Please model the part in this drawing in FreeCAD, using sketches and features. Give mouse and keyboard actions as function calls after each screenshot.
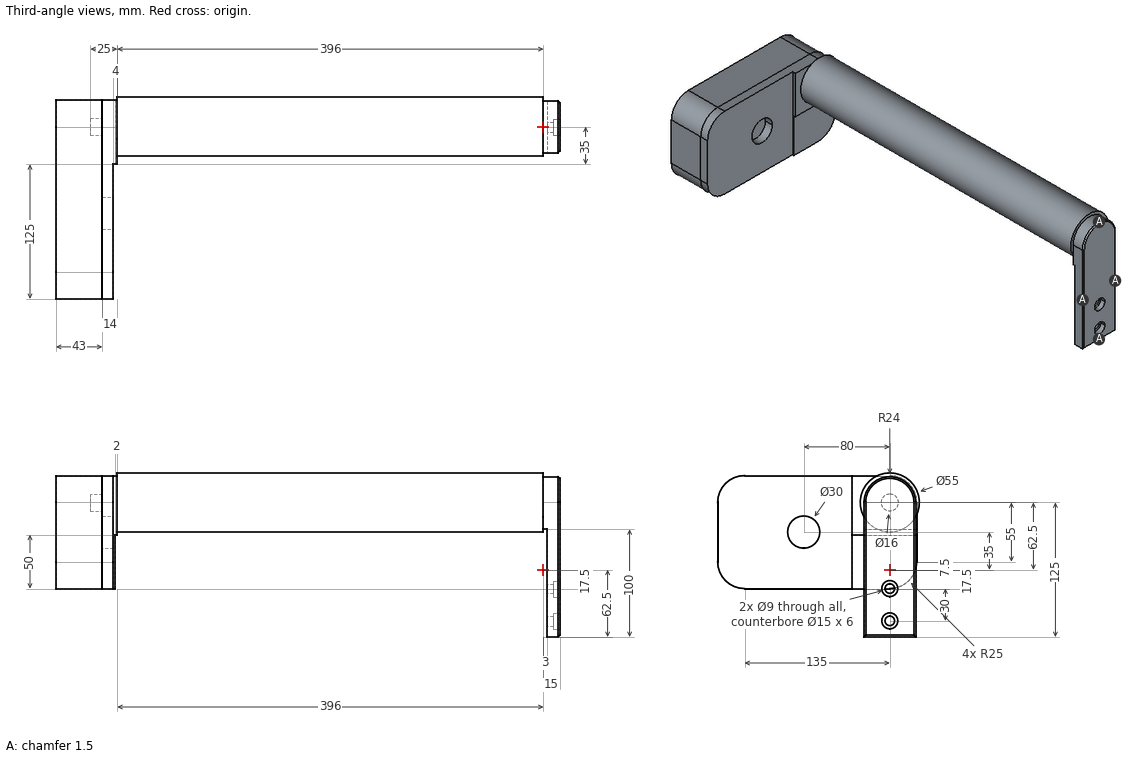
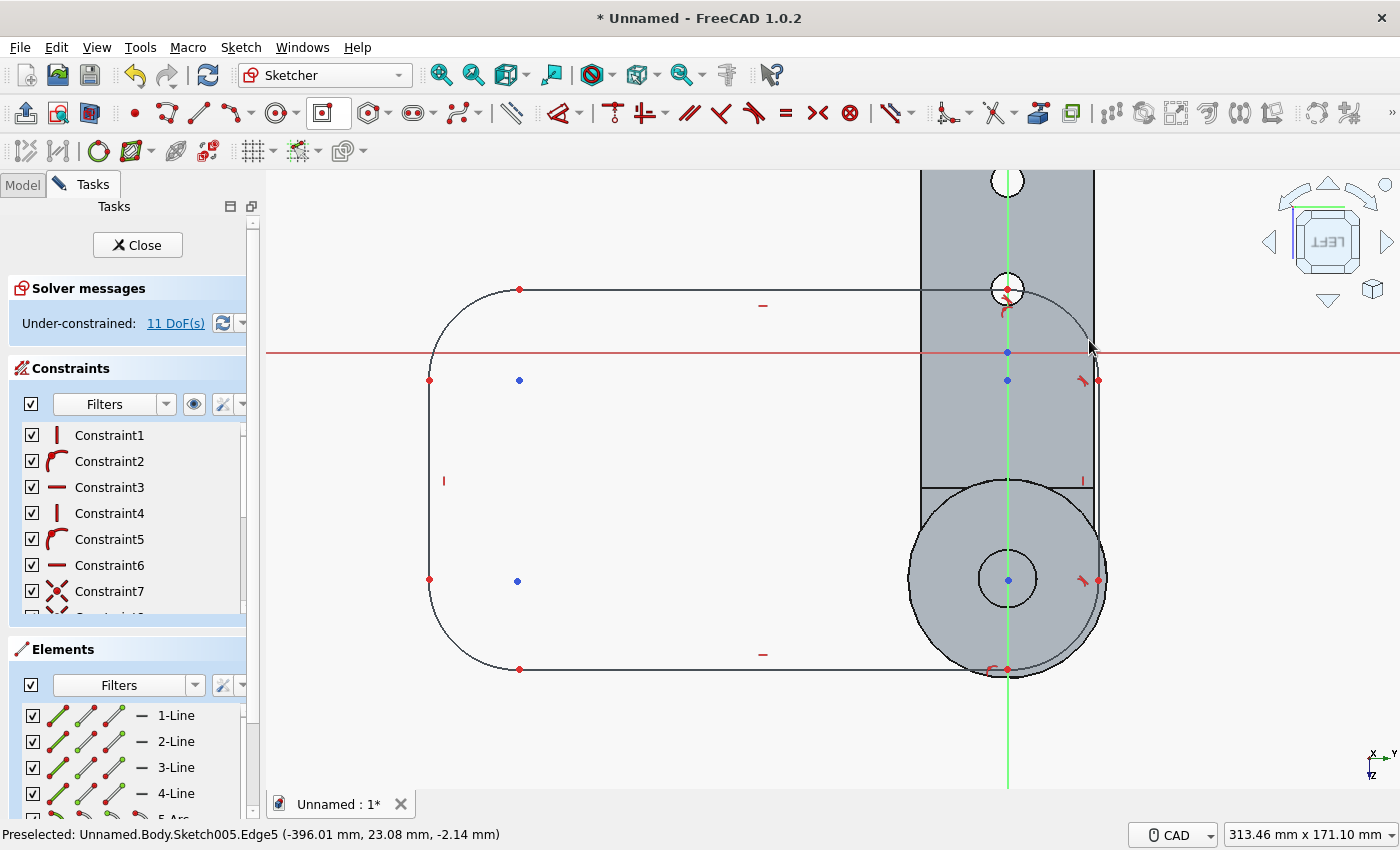
click(861, 290)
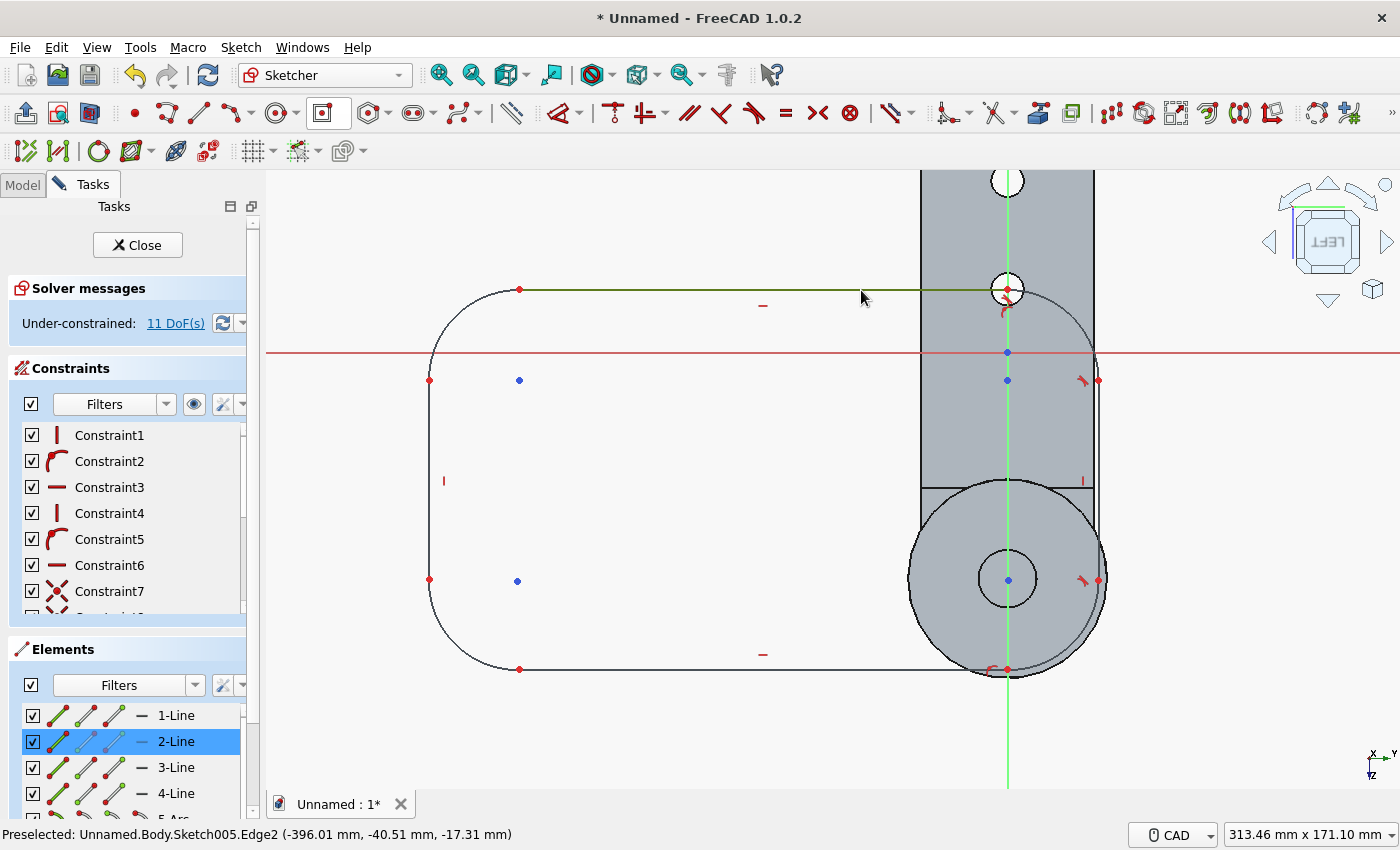
click(478, 300)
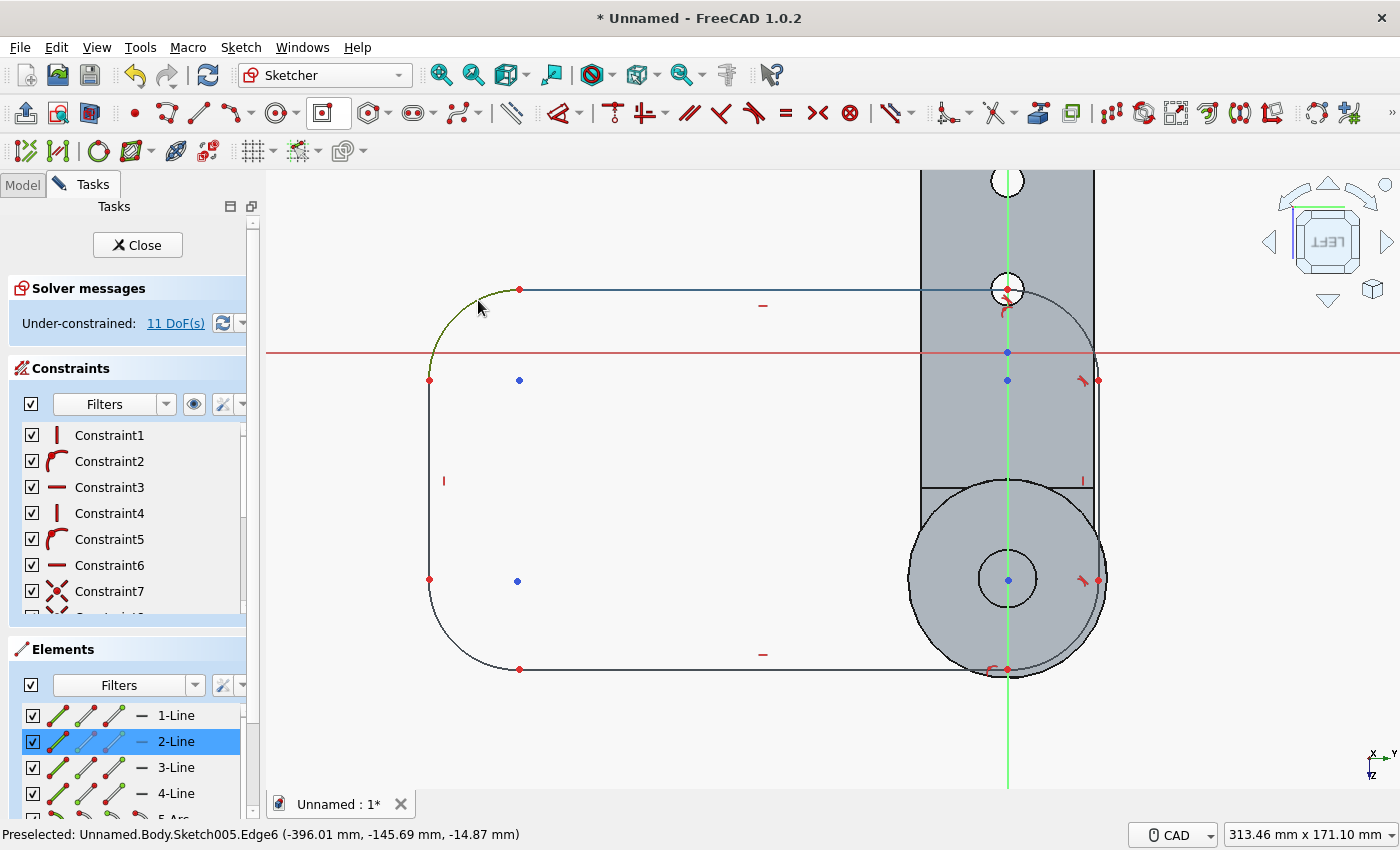
click(754, 114)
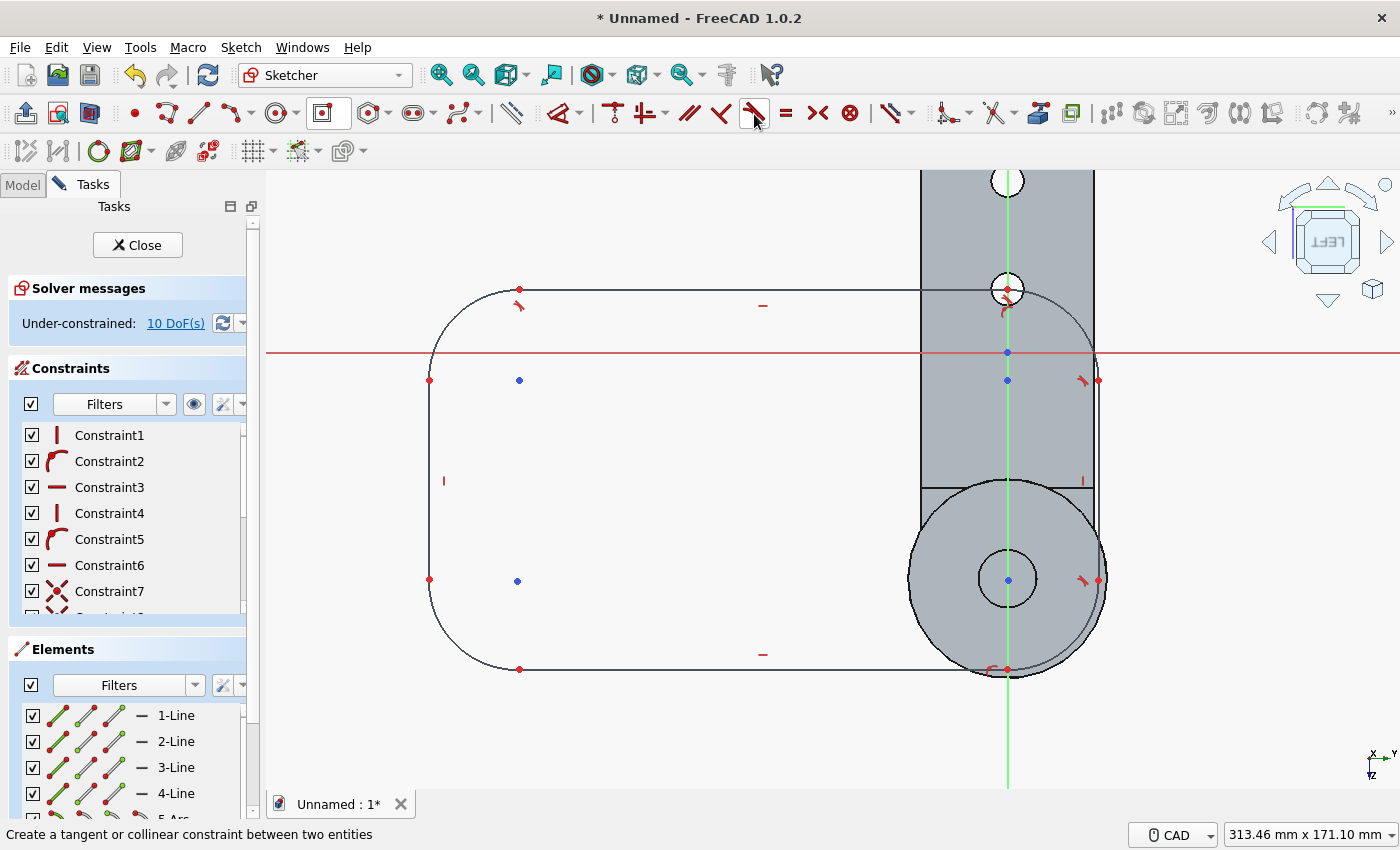
click(429, 441)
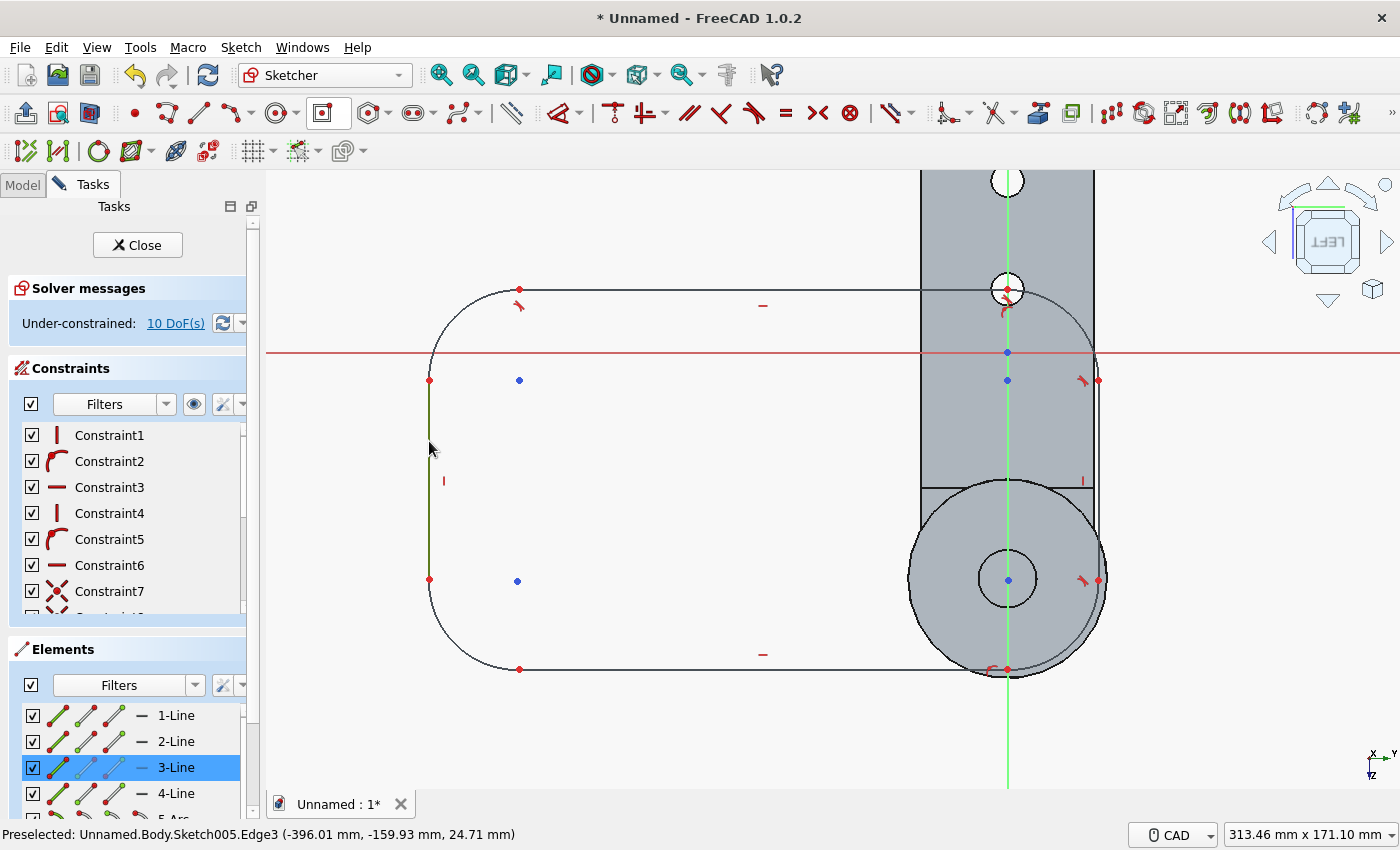
click(478, 300)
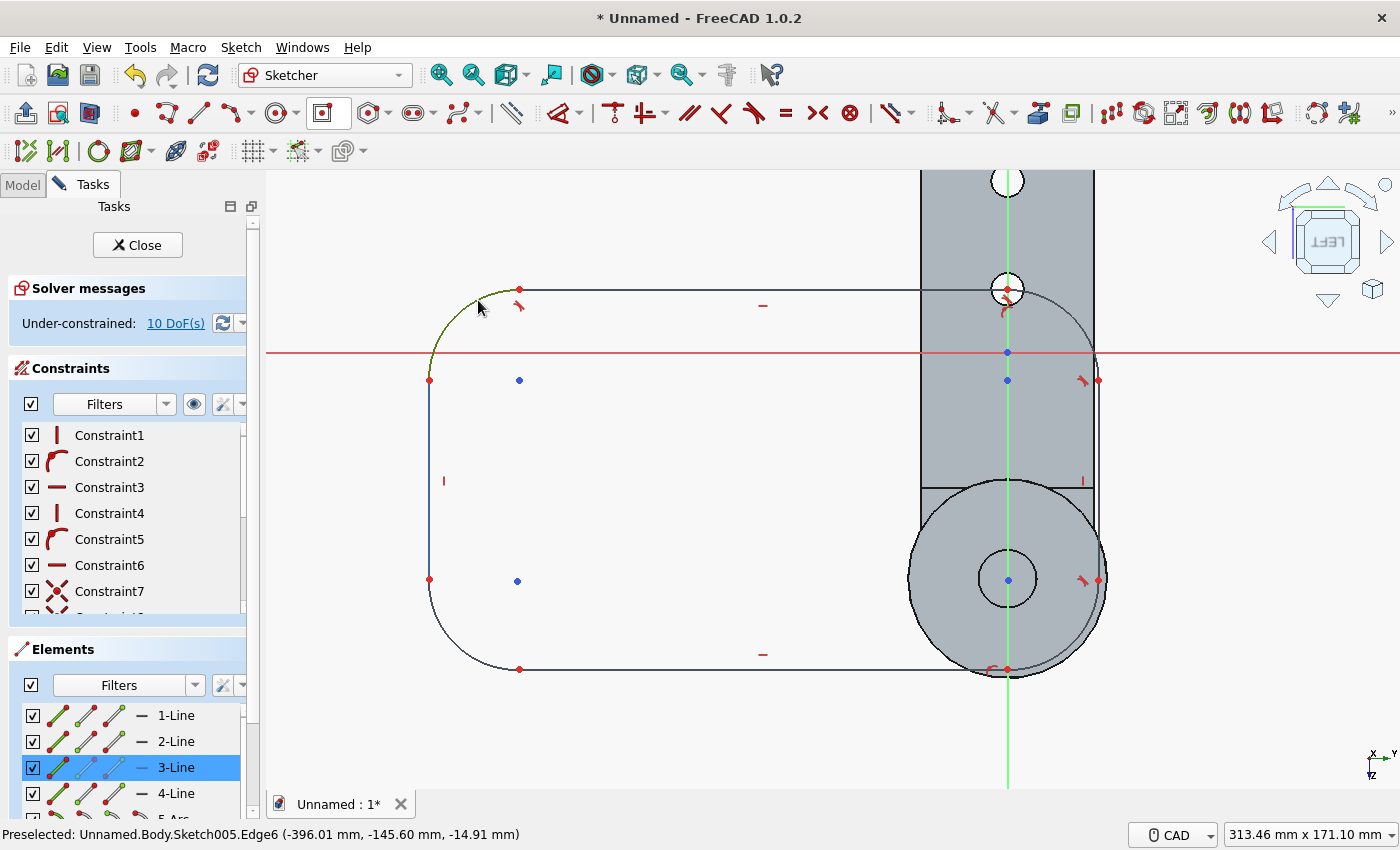
click(754, 114)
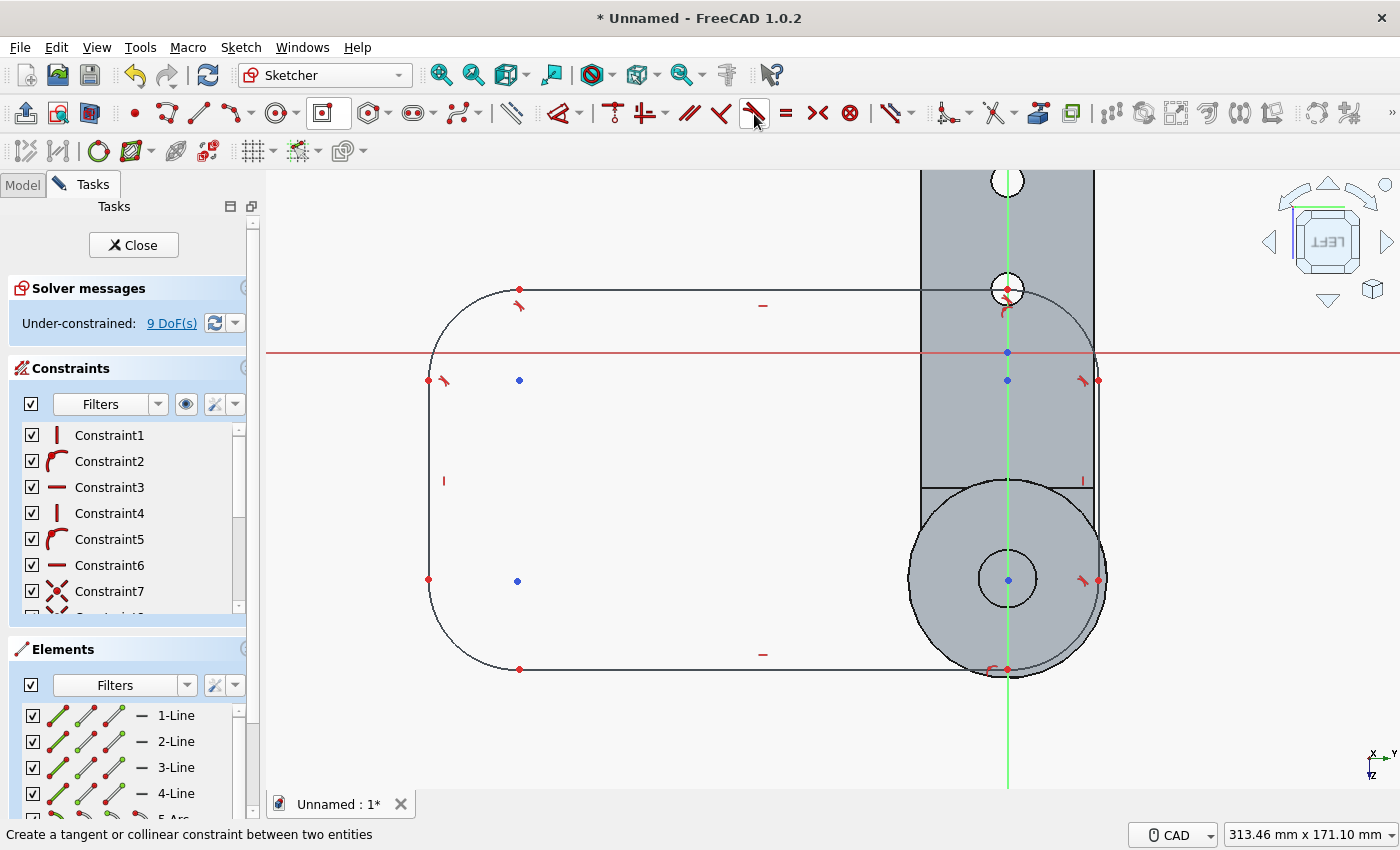
click(429, 441)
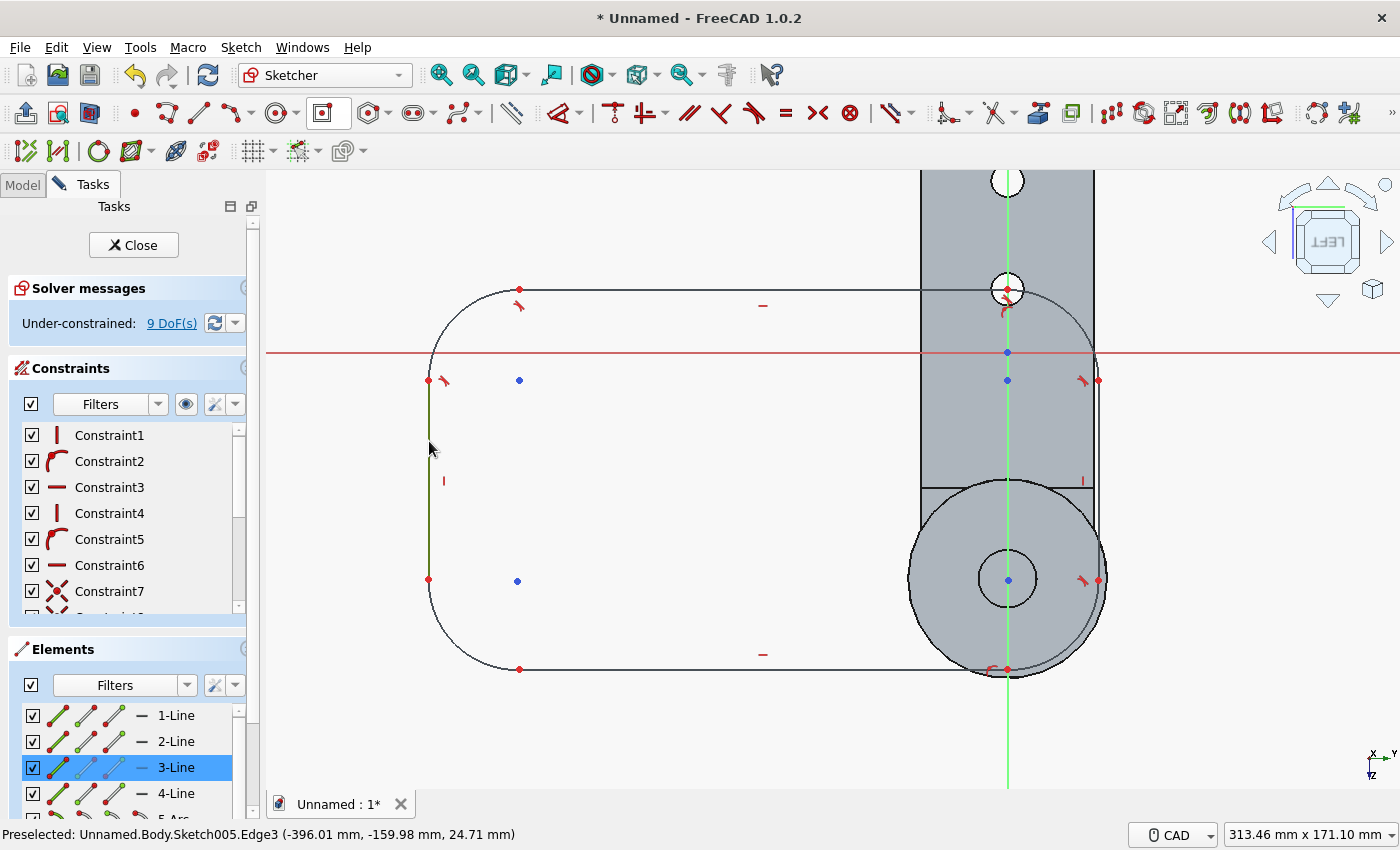
click(438, 621)